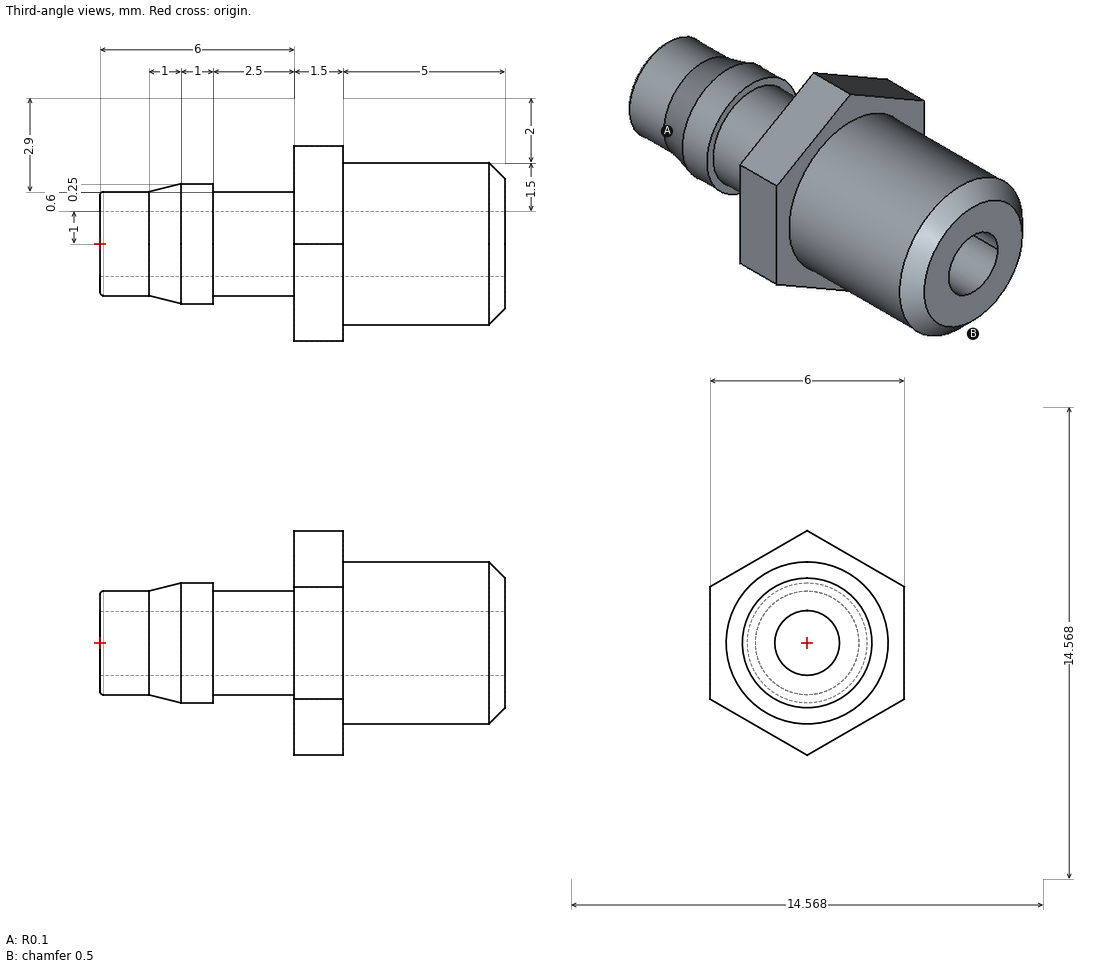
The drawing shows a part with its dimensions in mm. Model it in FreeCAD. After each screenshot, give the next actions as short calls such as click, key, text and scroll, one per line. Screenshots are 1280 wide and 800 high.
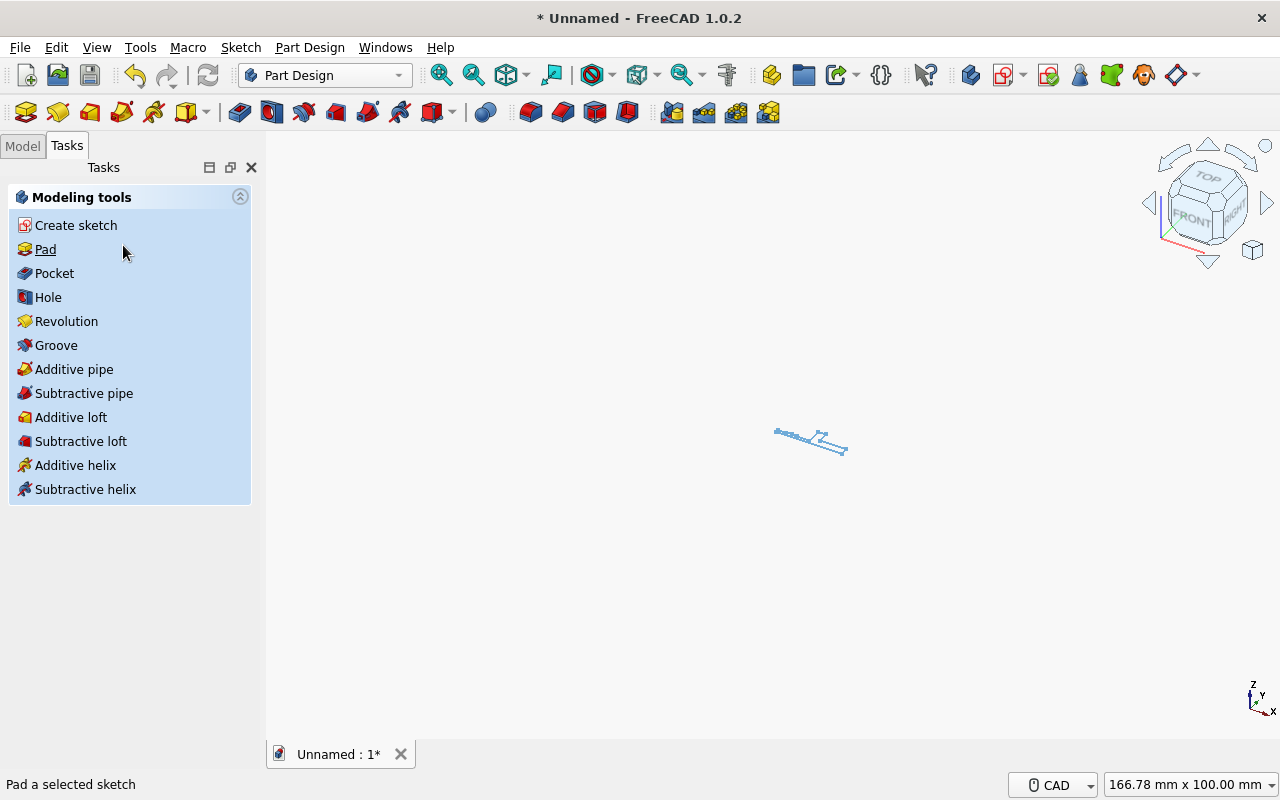
click(58, 112)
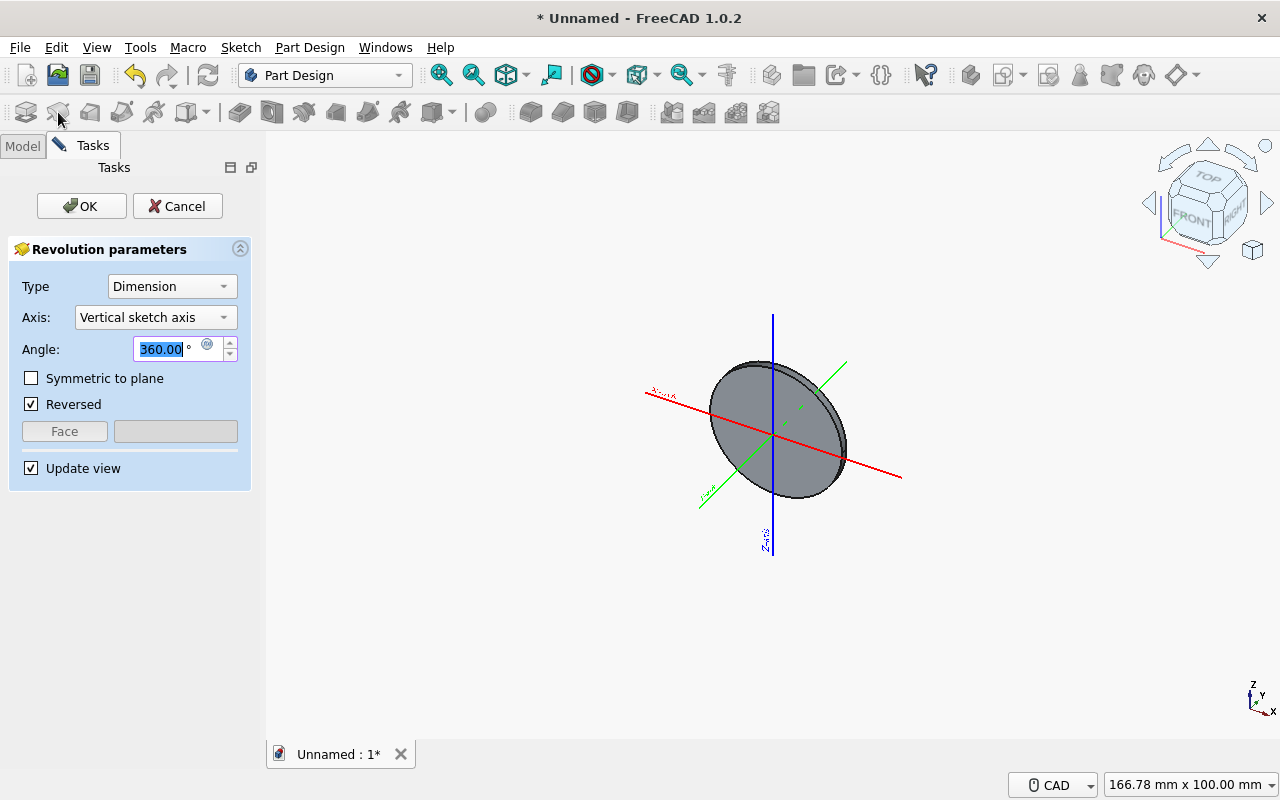
click(156, 318)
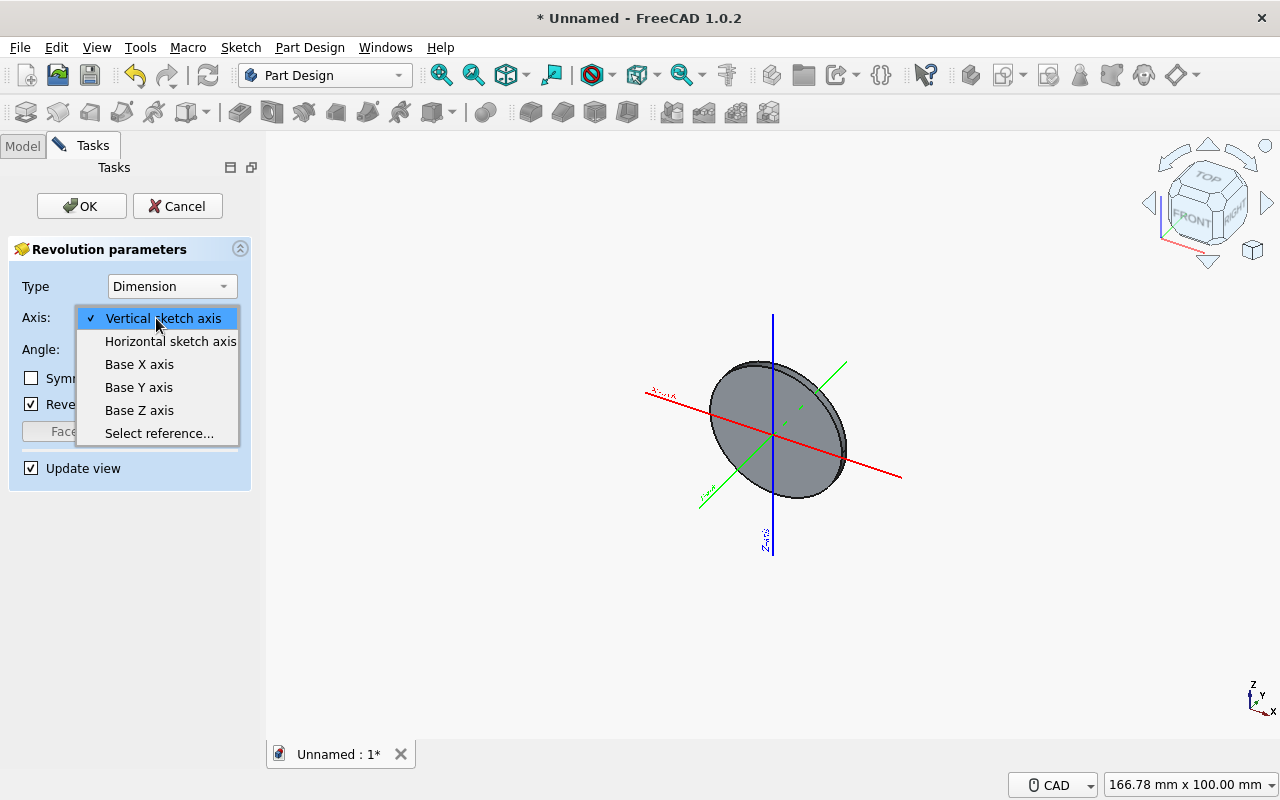
click(156, 342)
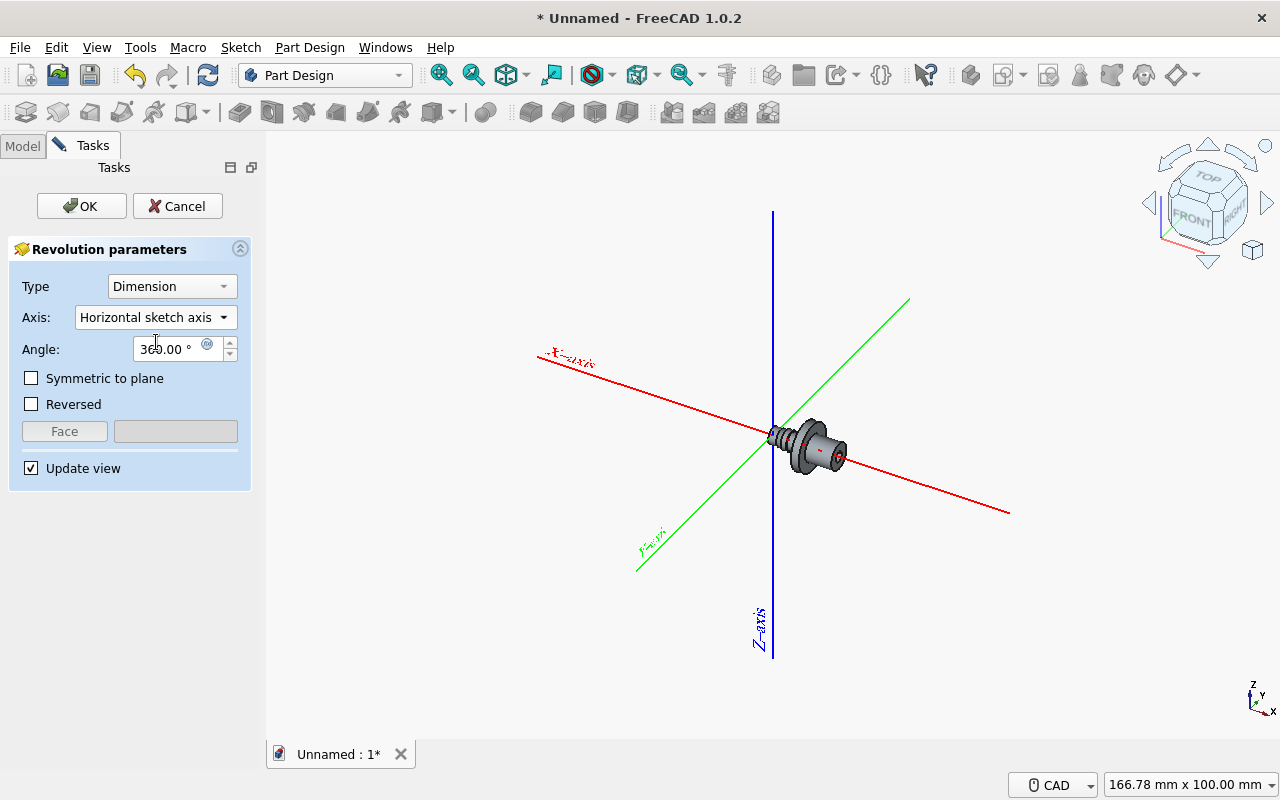
click(82, 206)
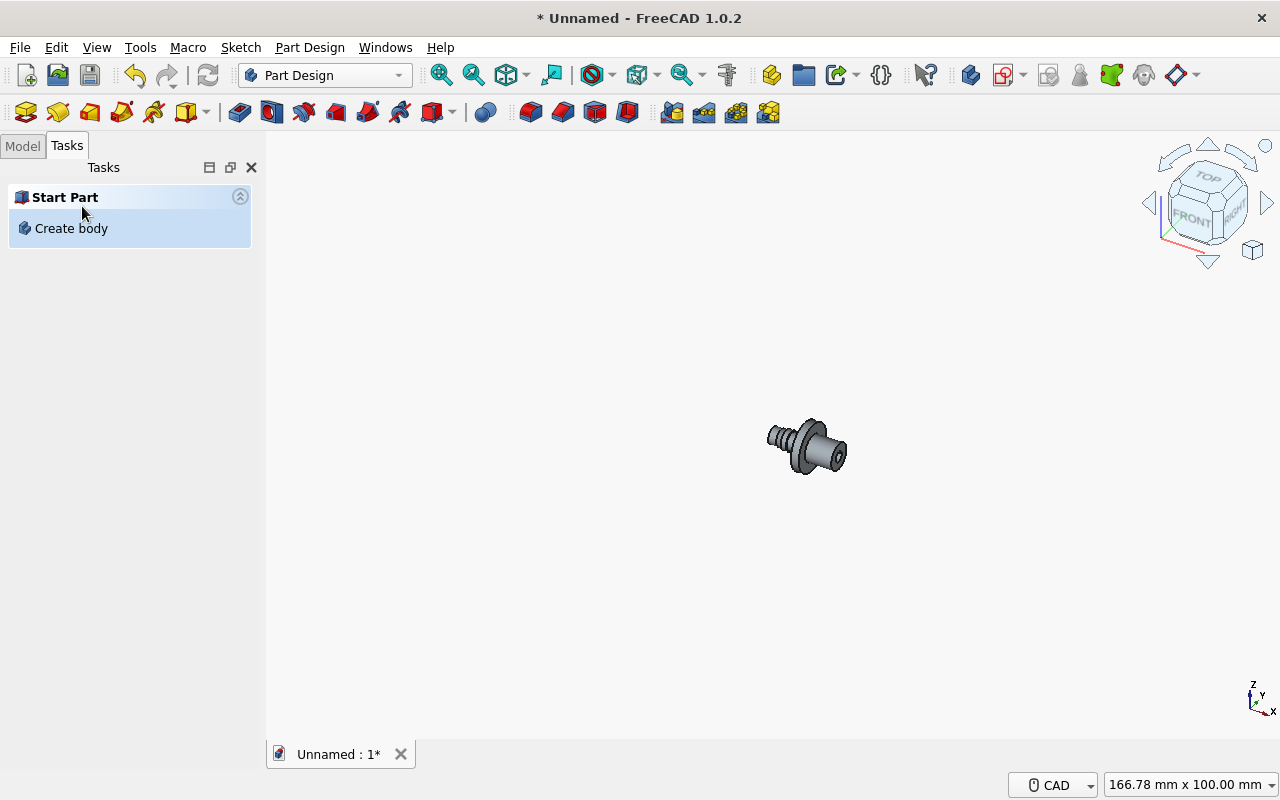
click(442, 76)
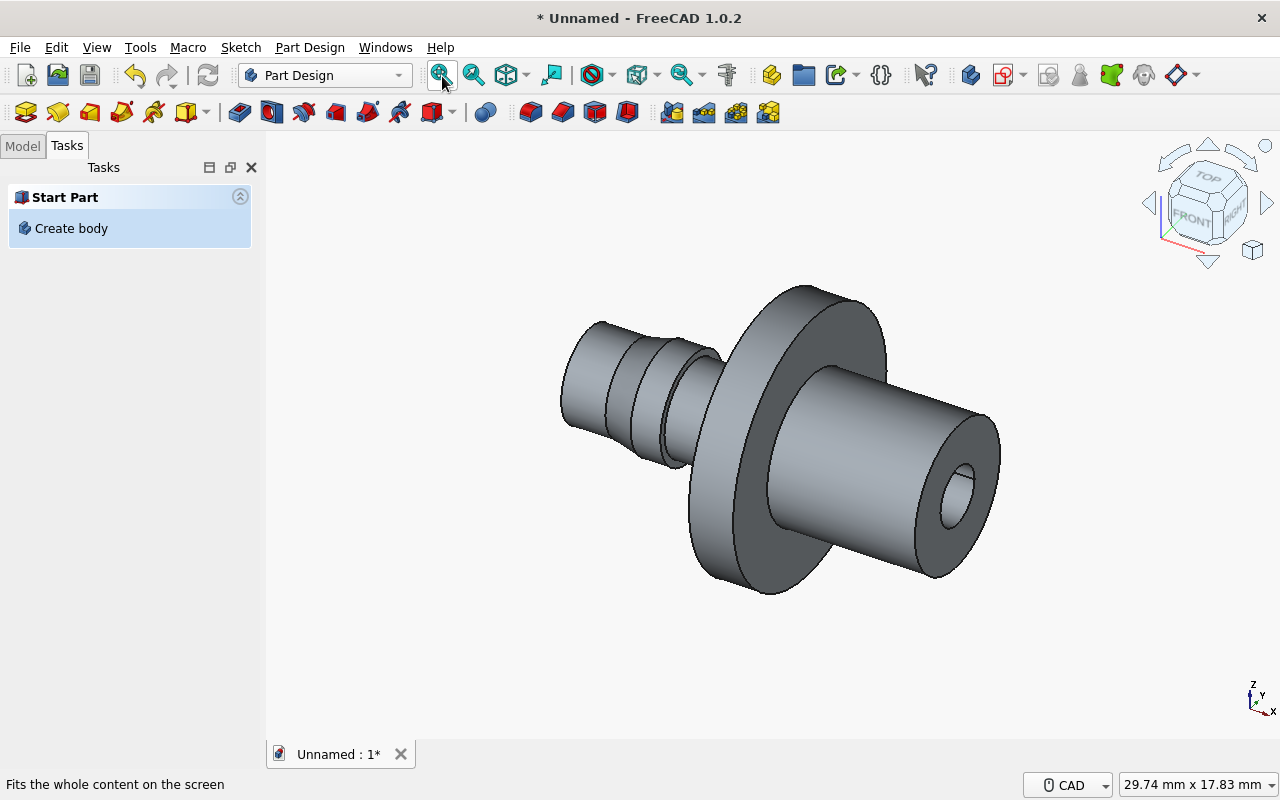
click(766, 562)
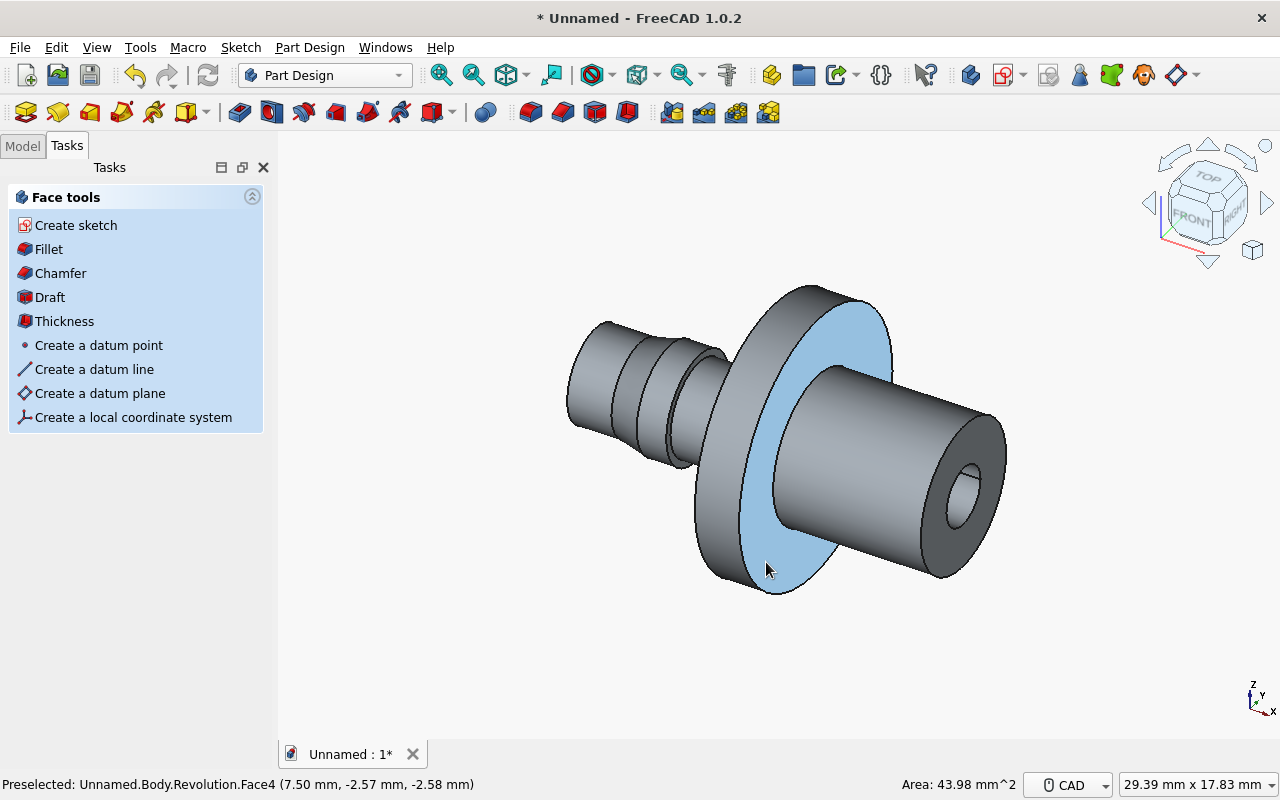
click(1004, 76)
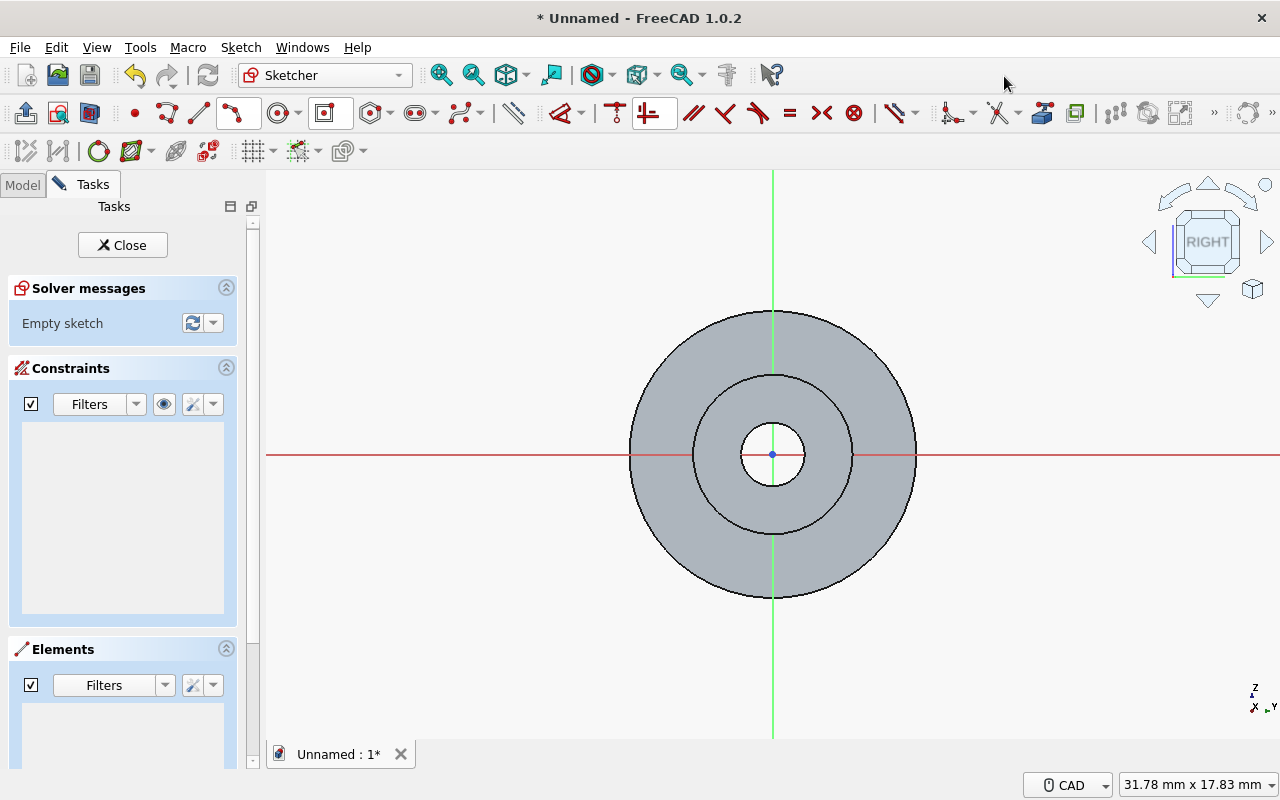
scroll(396, 455, down, 1)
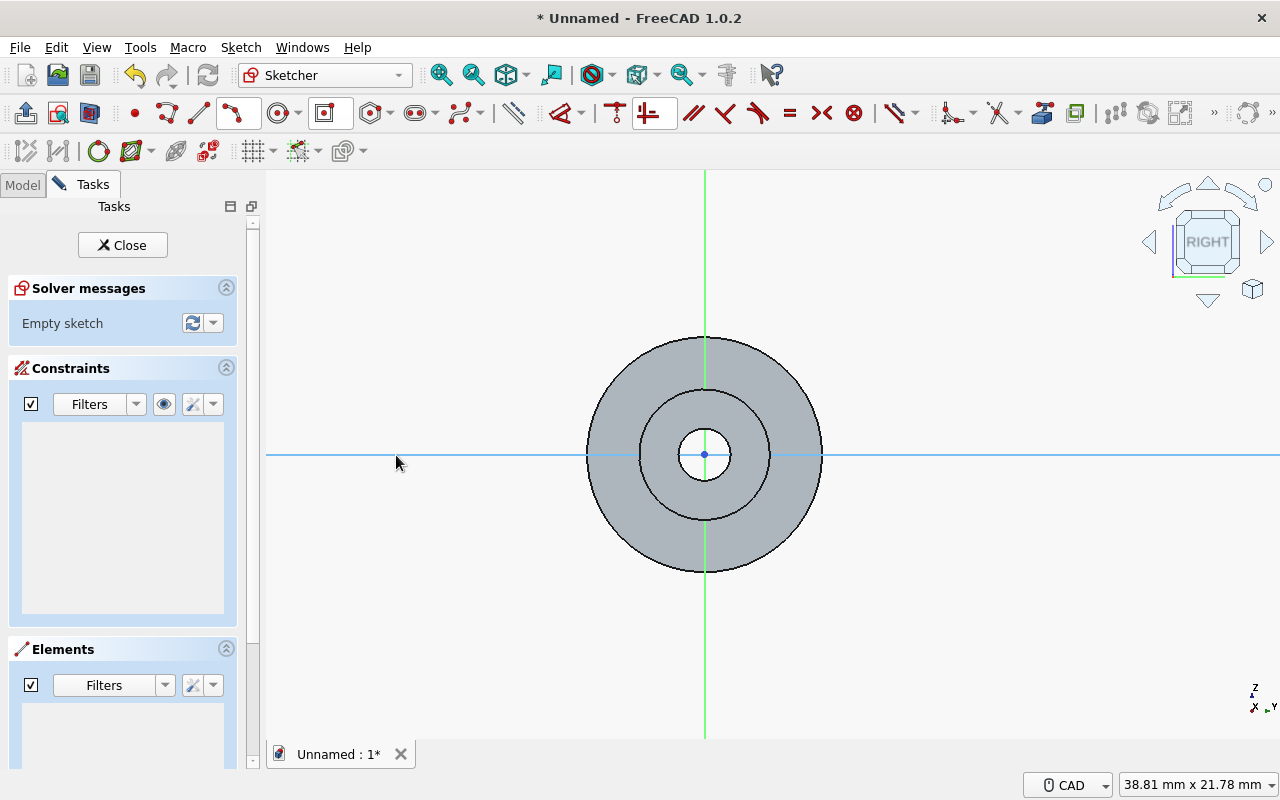
click(324, 114)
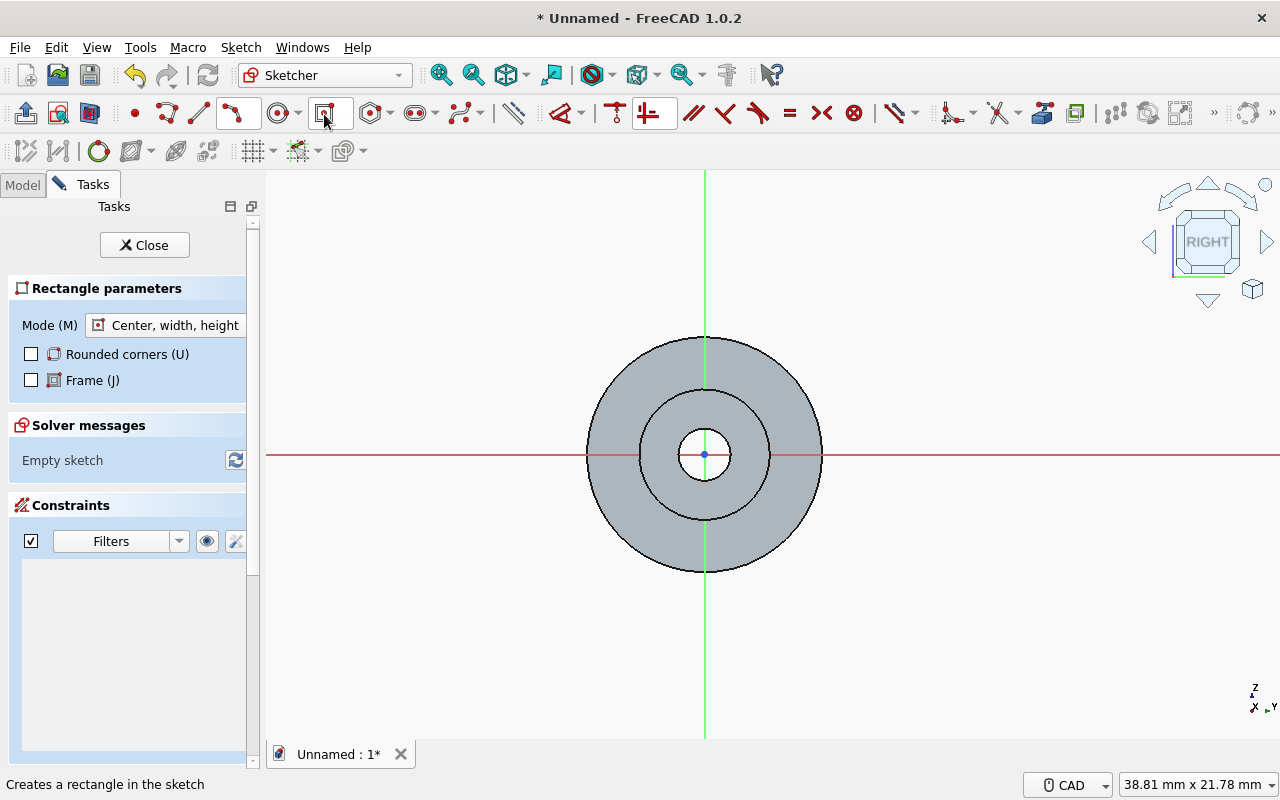
click(705, 455)
move(895, 264)